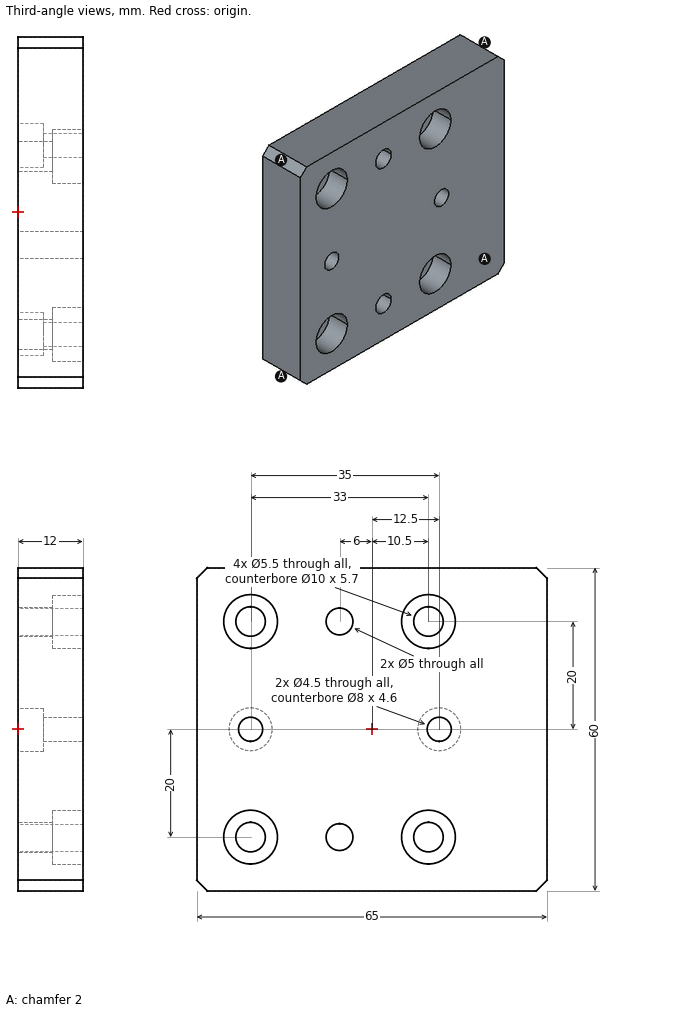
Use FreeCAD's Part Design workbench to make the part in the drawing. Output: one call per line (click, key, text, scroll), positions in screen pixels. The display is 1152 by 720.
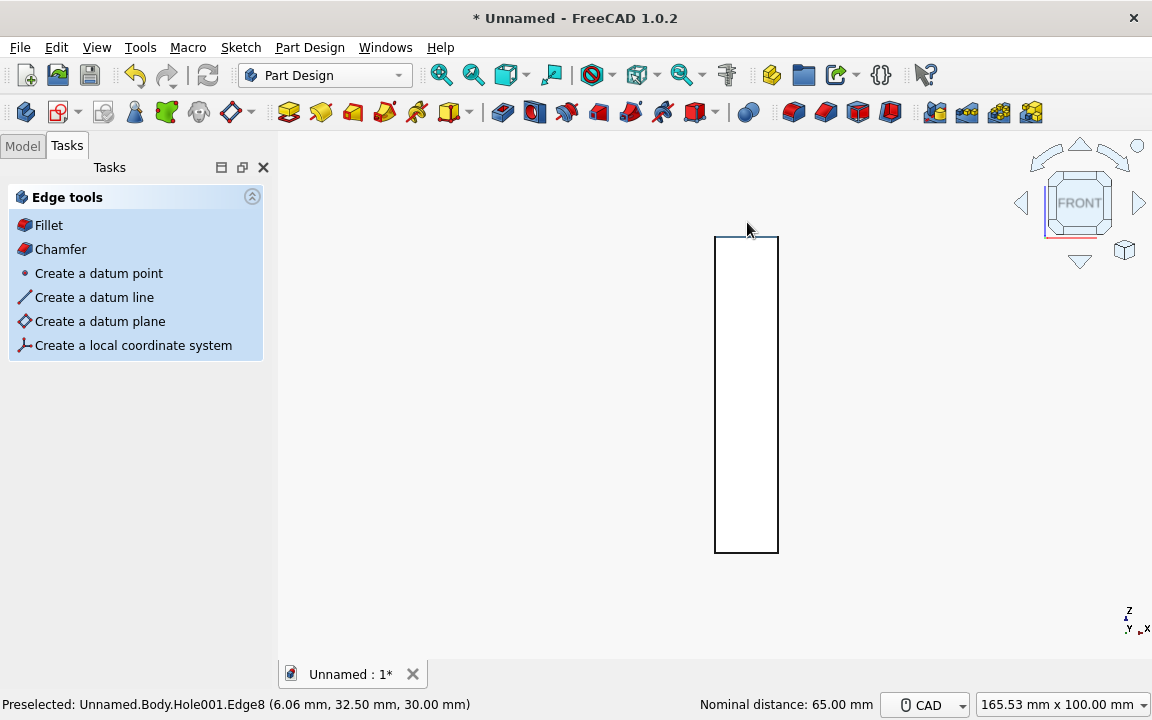
click(747, 552, ctrl)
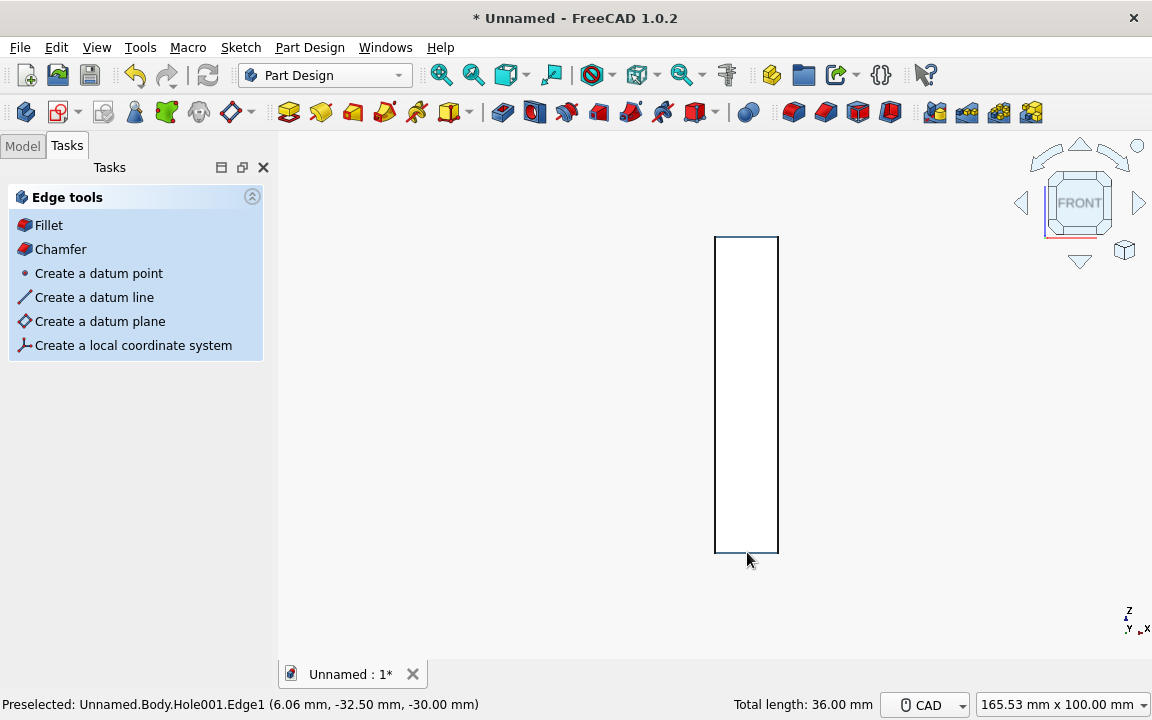
key(3)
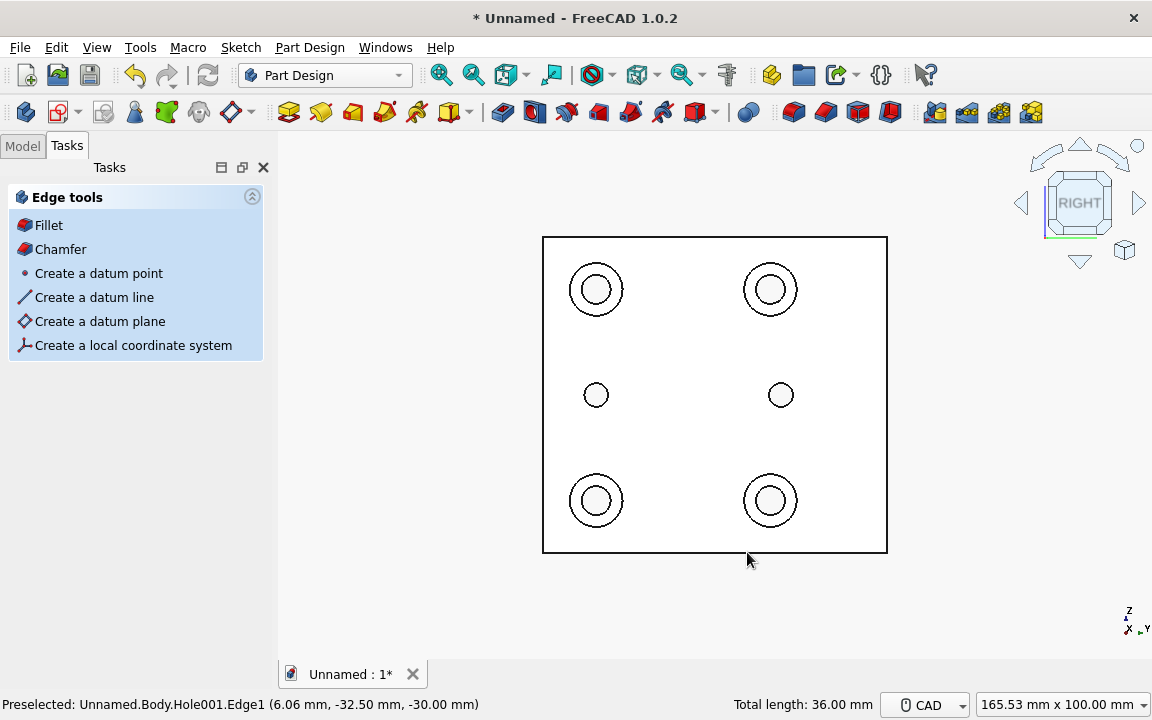
key(5)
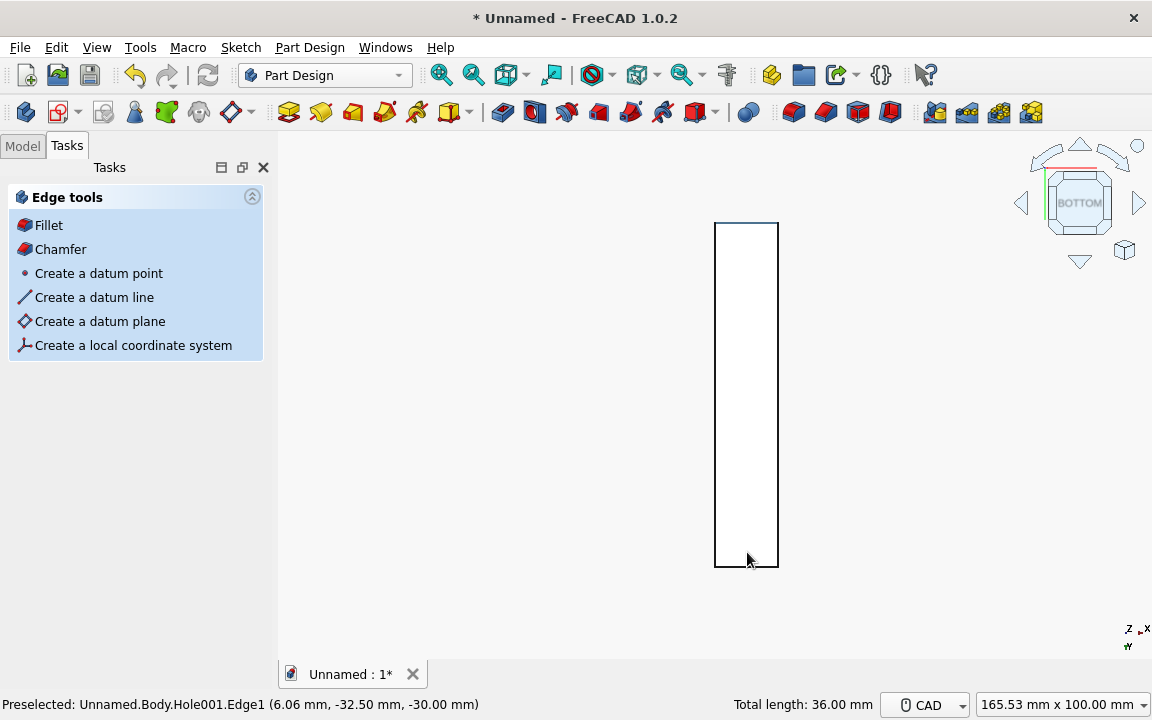
click(747, 566, ctrl)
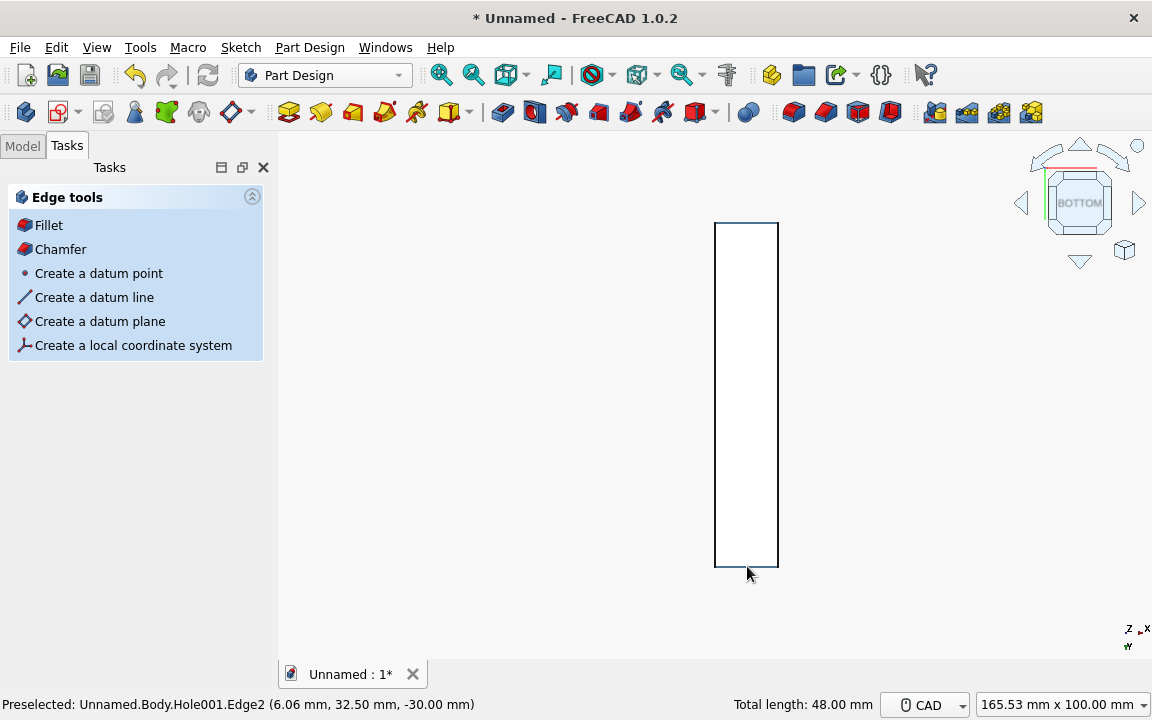
click(826, 112)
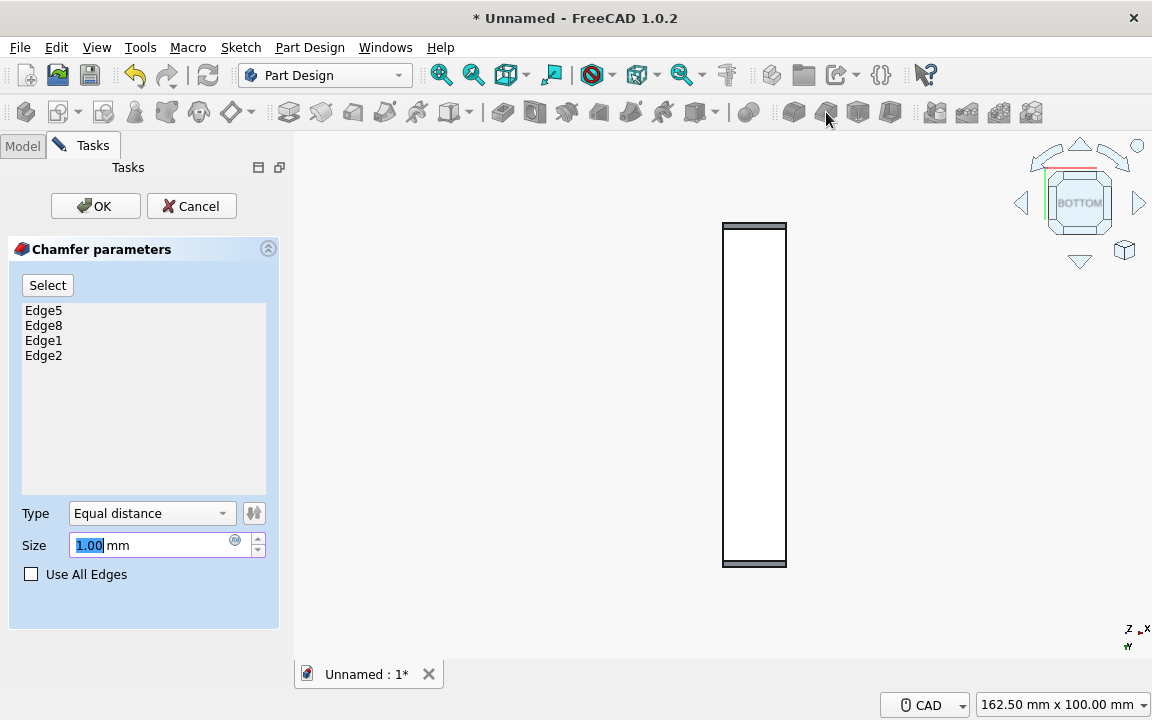
text(2)
key(Tab)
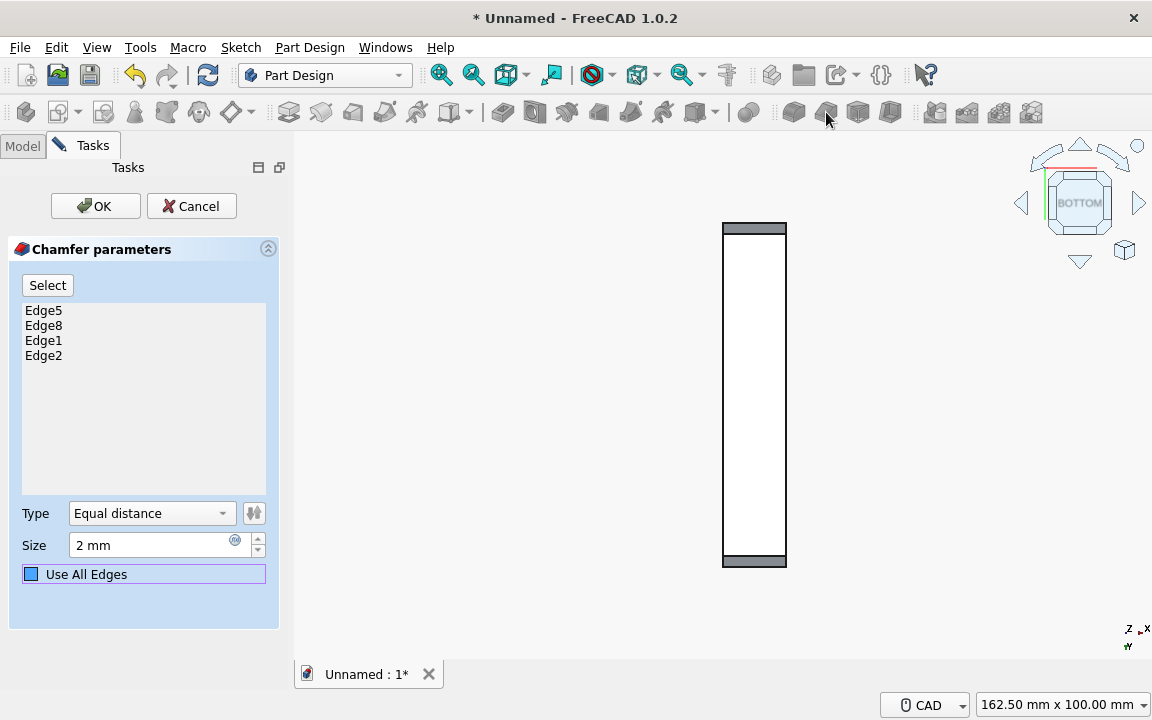
click(96, 206)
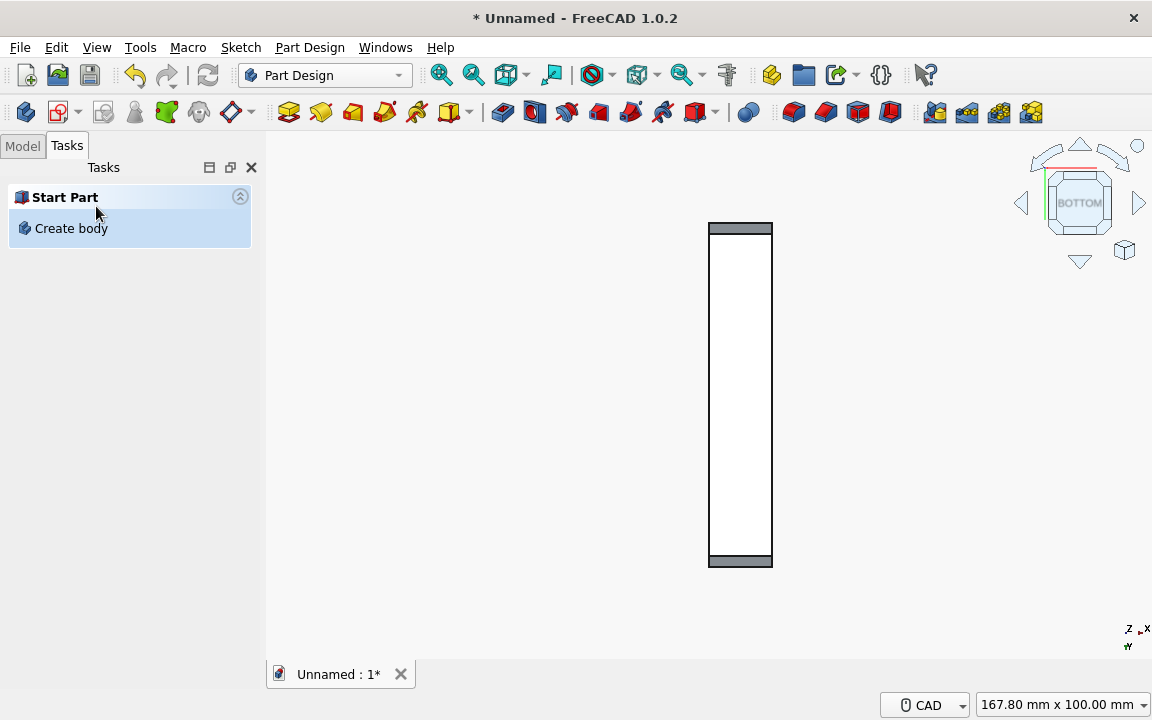
key(0)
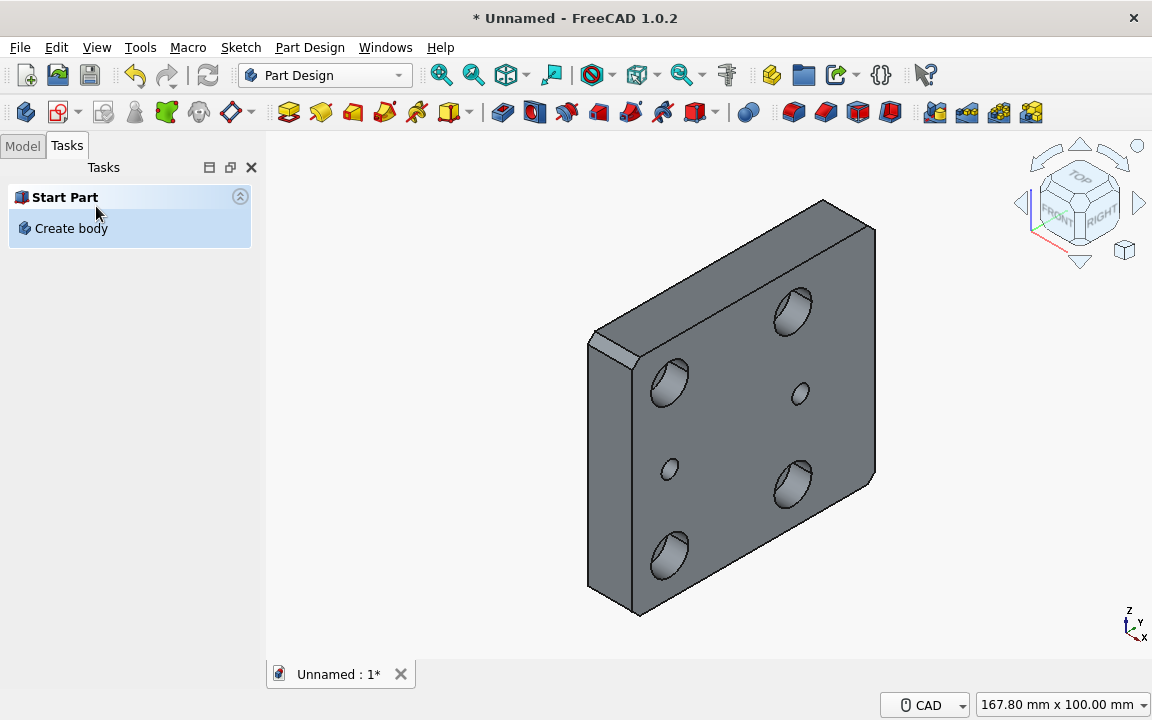
click(719, 403)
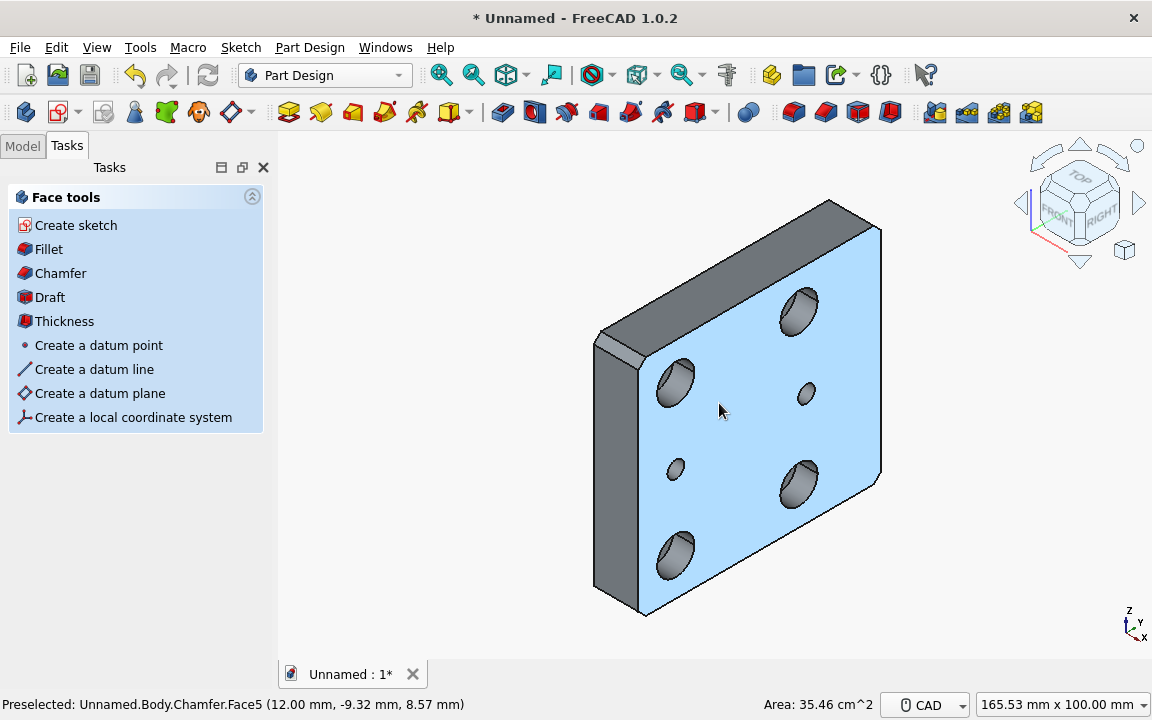
click(58, 112)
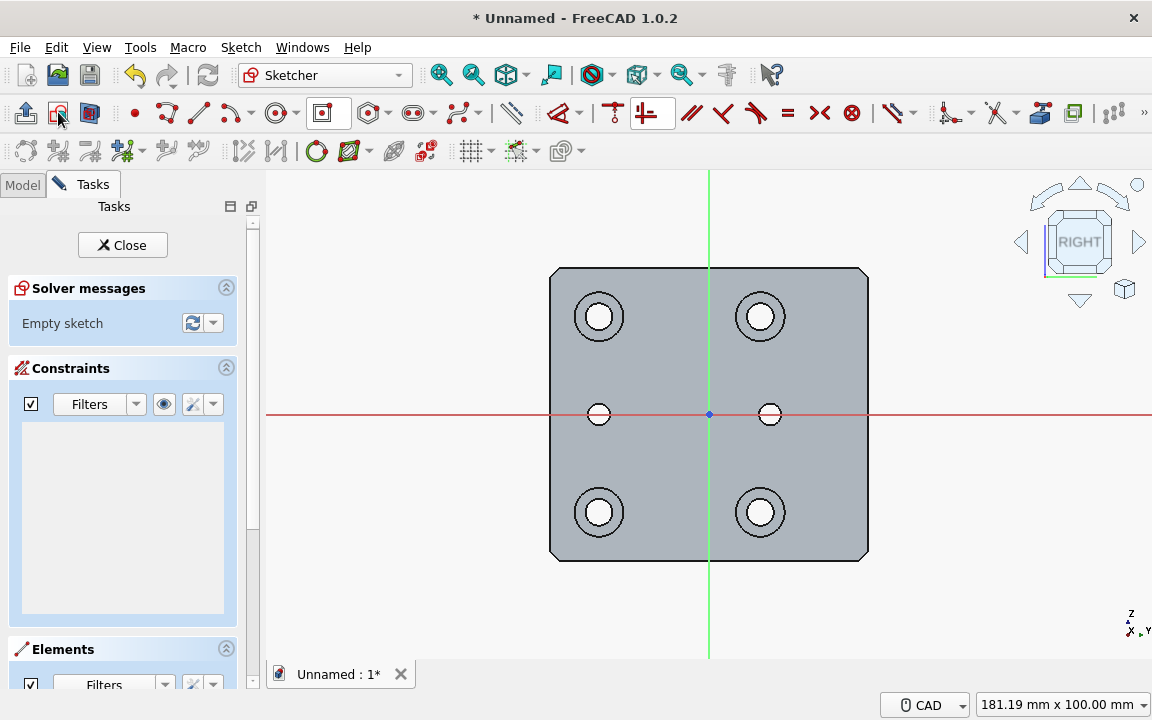
scroll(785, 414, up, 2)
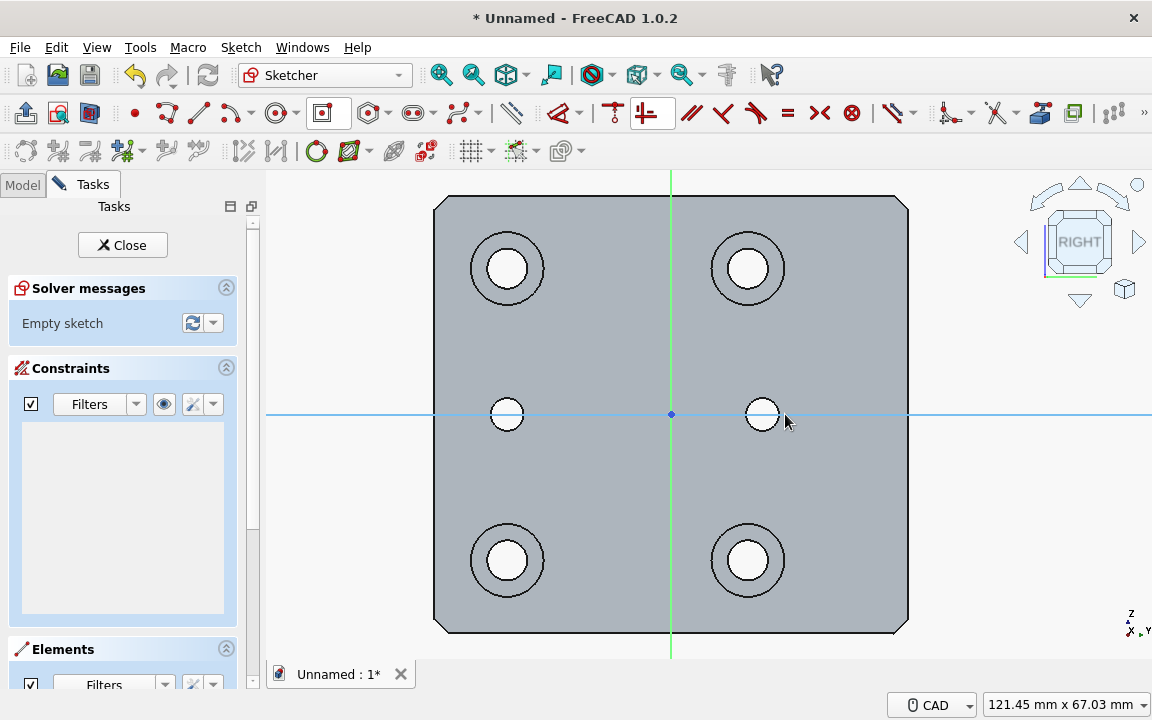
click(276, 114)